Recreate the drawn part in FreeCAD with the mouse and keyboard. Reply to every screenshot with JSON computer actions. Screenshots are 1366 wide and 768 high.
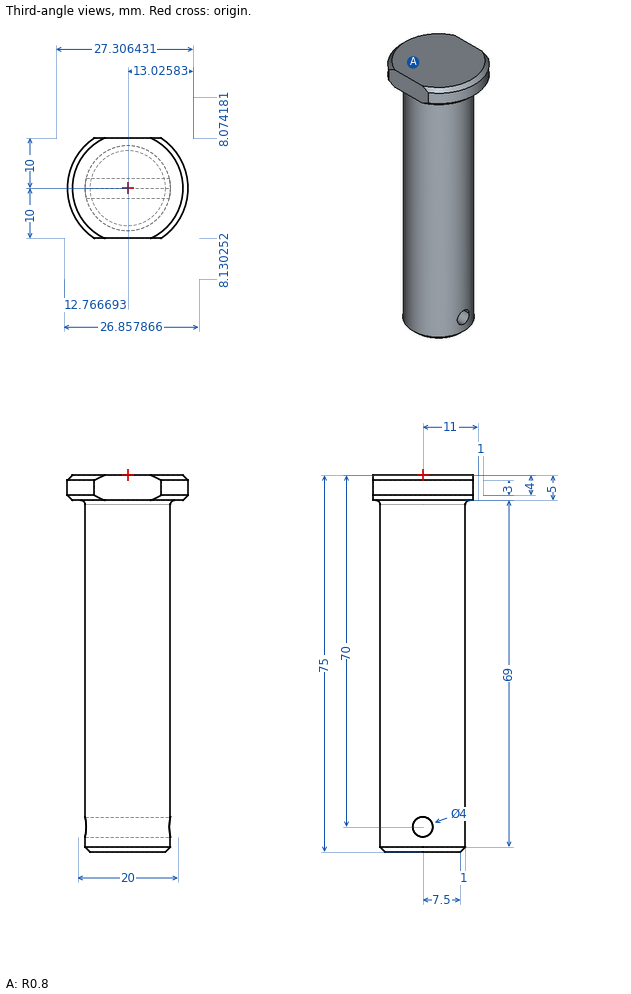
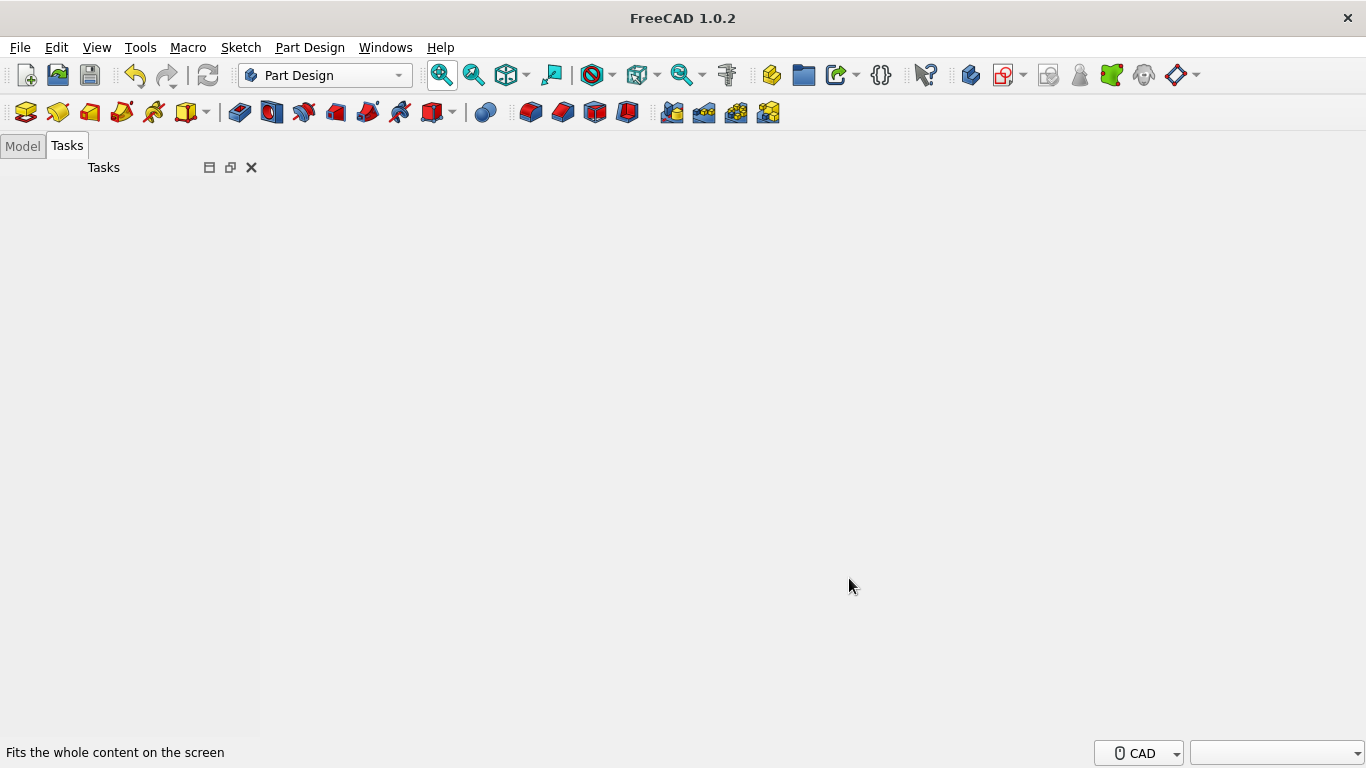
{"action": "left_click", "coordinate": [26, 76]}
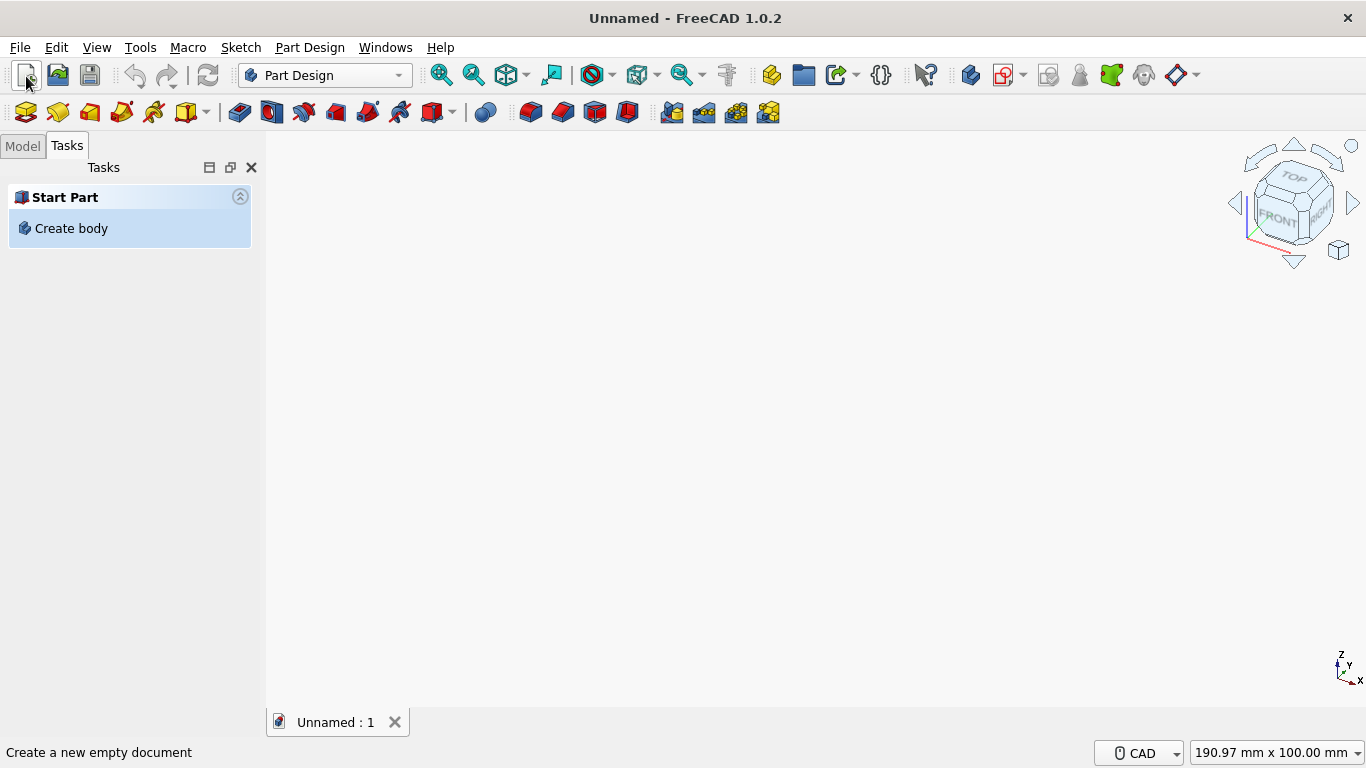
{"action": "left_click", "coordinate": [1004, 76]}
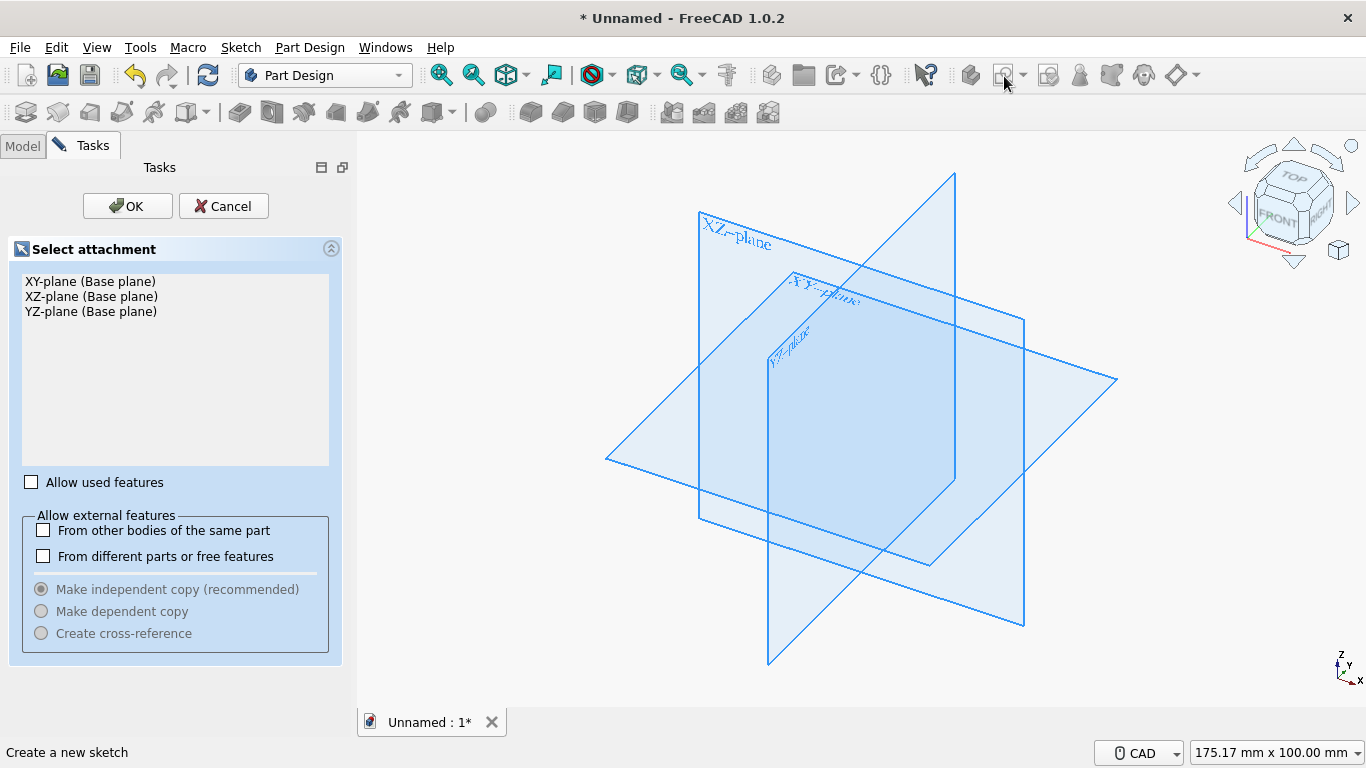
{"action": "left_click", "coordinate": [82, 312]}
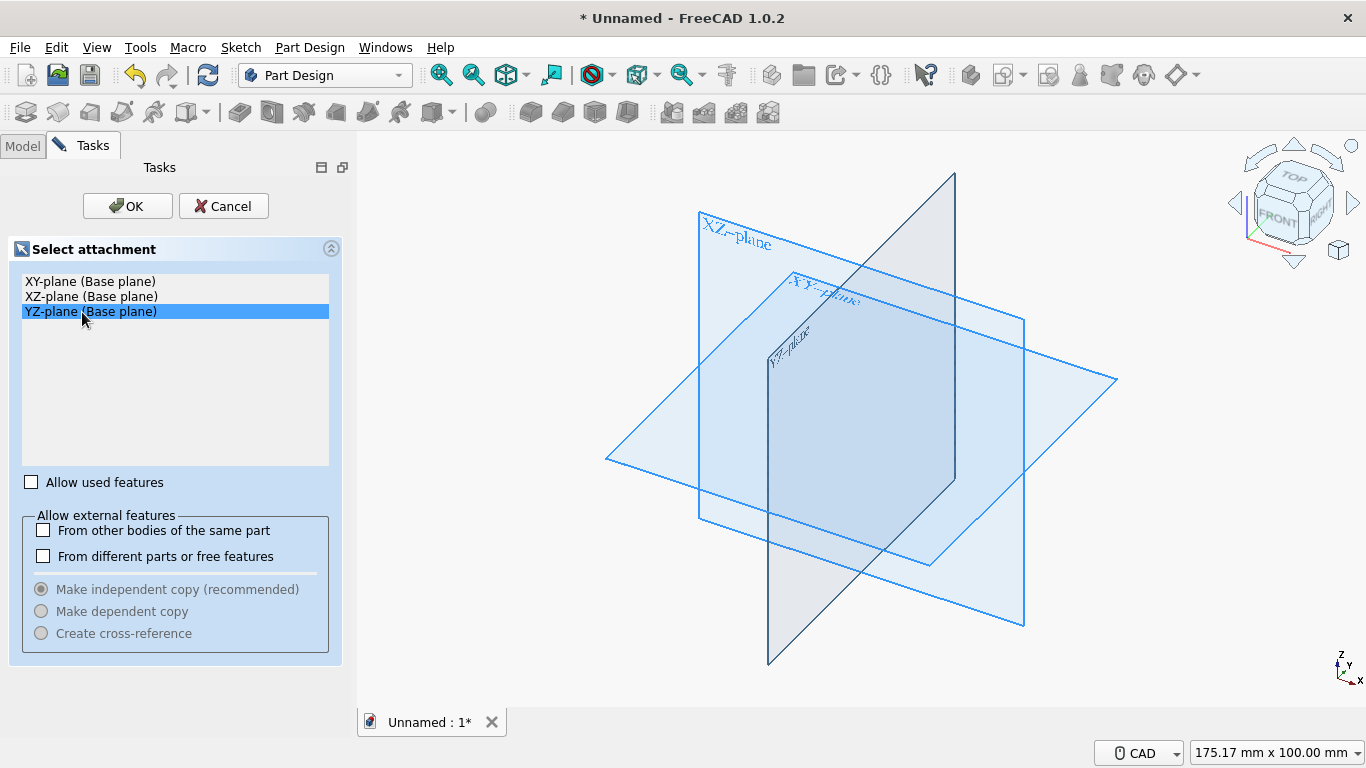
{"action": "left_click", "coordinate": [128, 206]}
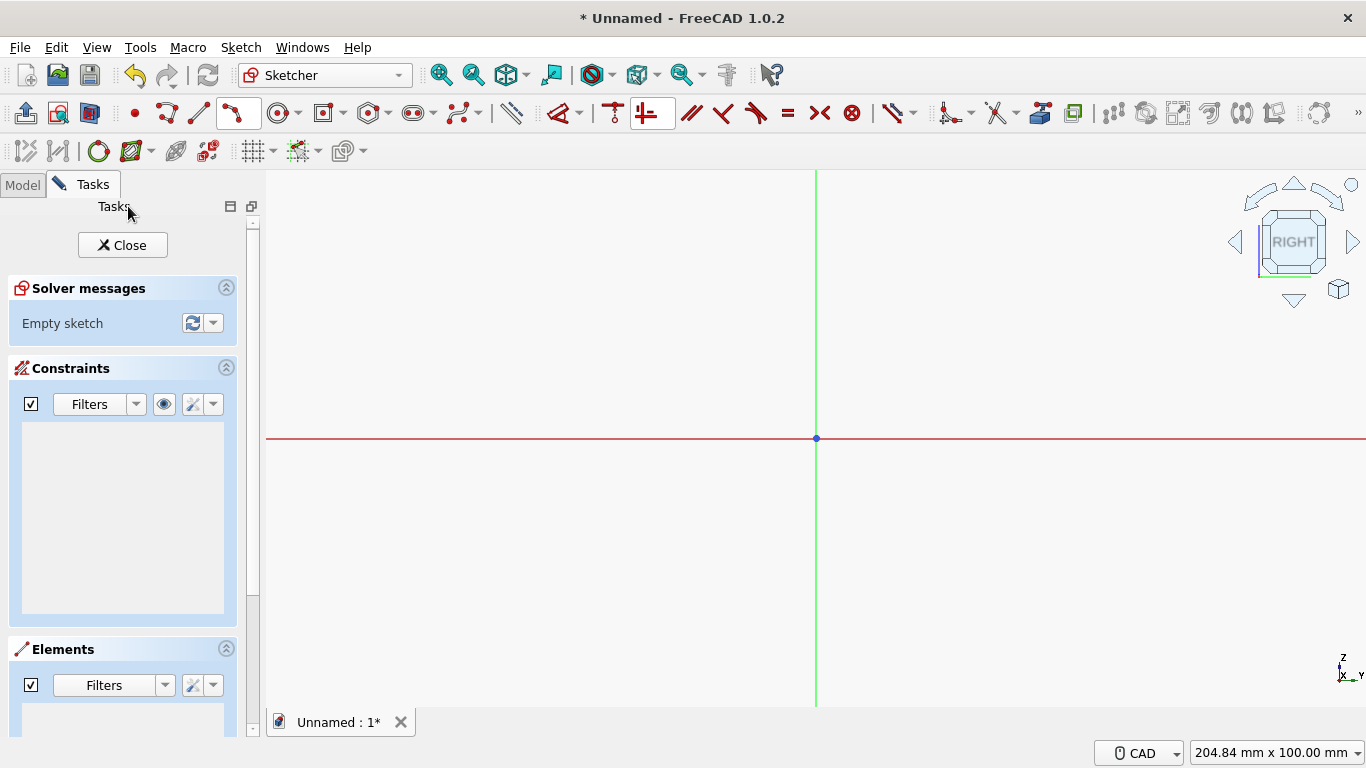
{"action": "scroll", "coordinate": [543, 198], "scroll_direction": "down", "scroll_amount": 2}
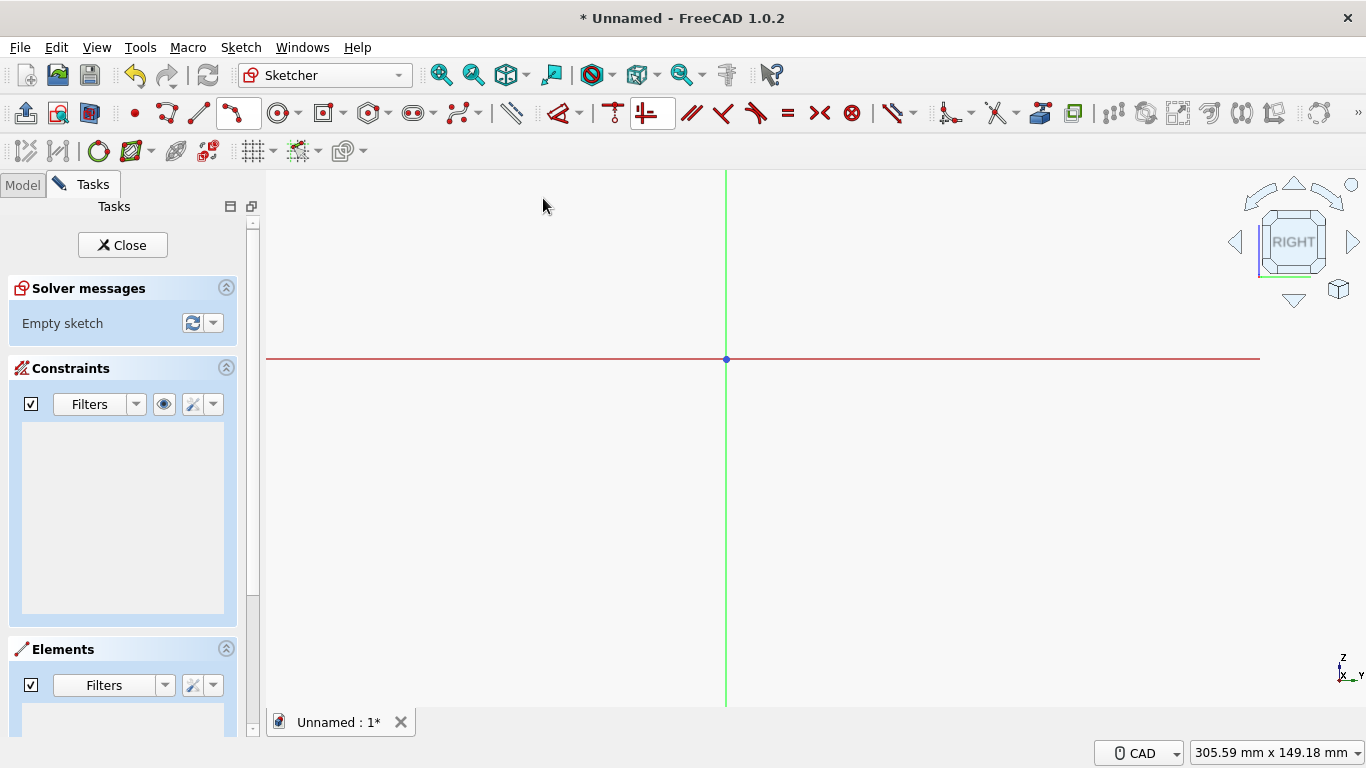
{"action": "left_click", "coordinate": [168, 114]}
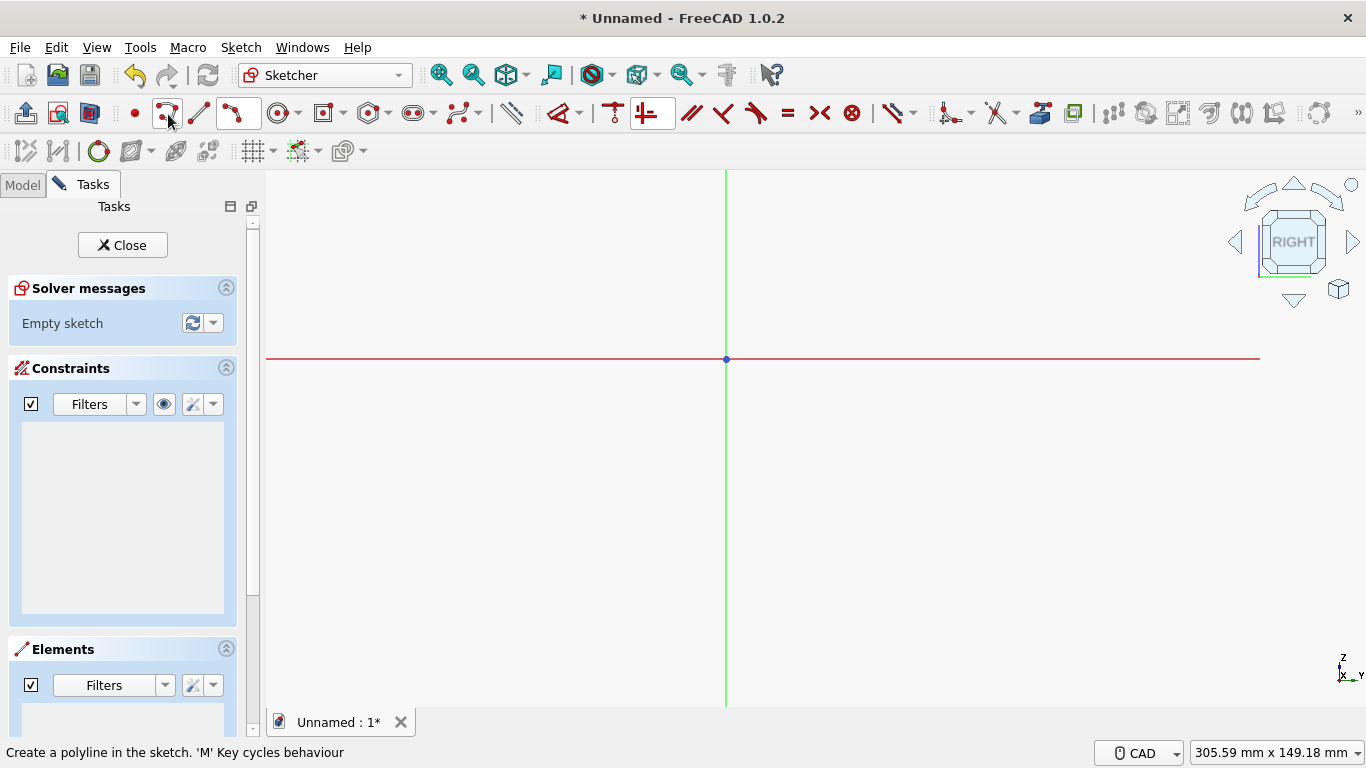
{"action": "left_click", "coordinate": [726, 359]}
{"action": "left_click", "coordinate": [735, 629]}
{"action": "left_click", "coordinate": [753, 629]}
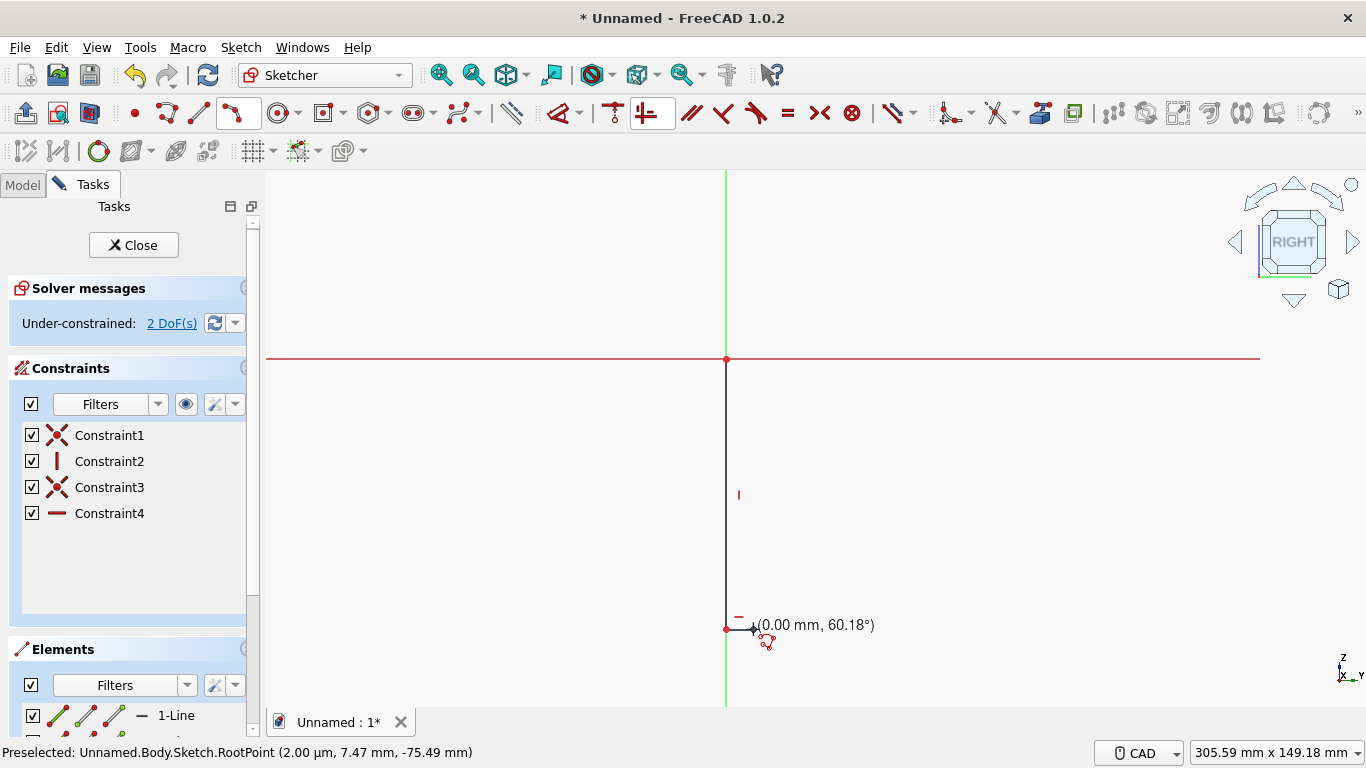
{"action": "scroll", "coordinate": [757, 626], "scroll_direction": "up", "scroll_amount": 6}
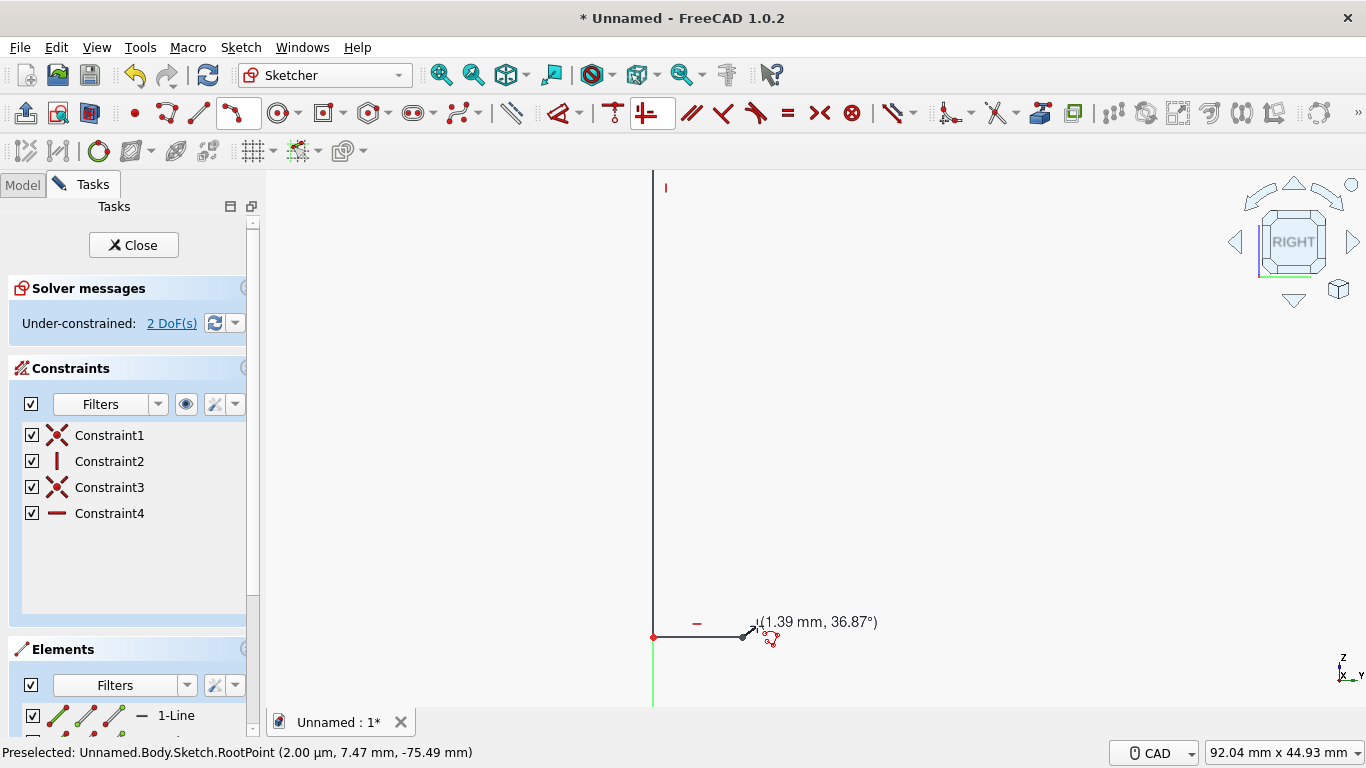
{"action": "left_click", "coordinate": [755, 623]}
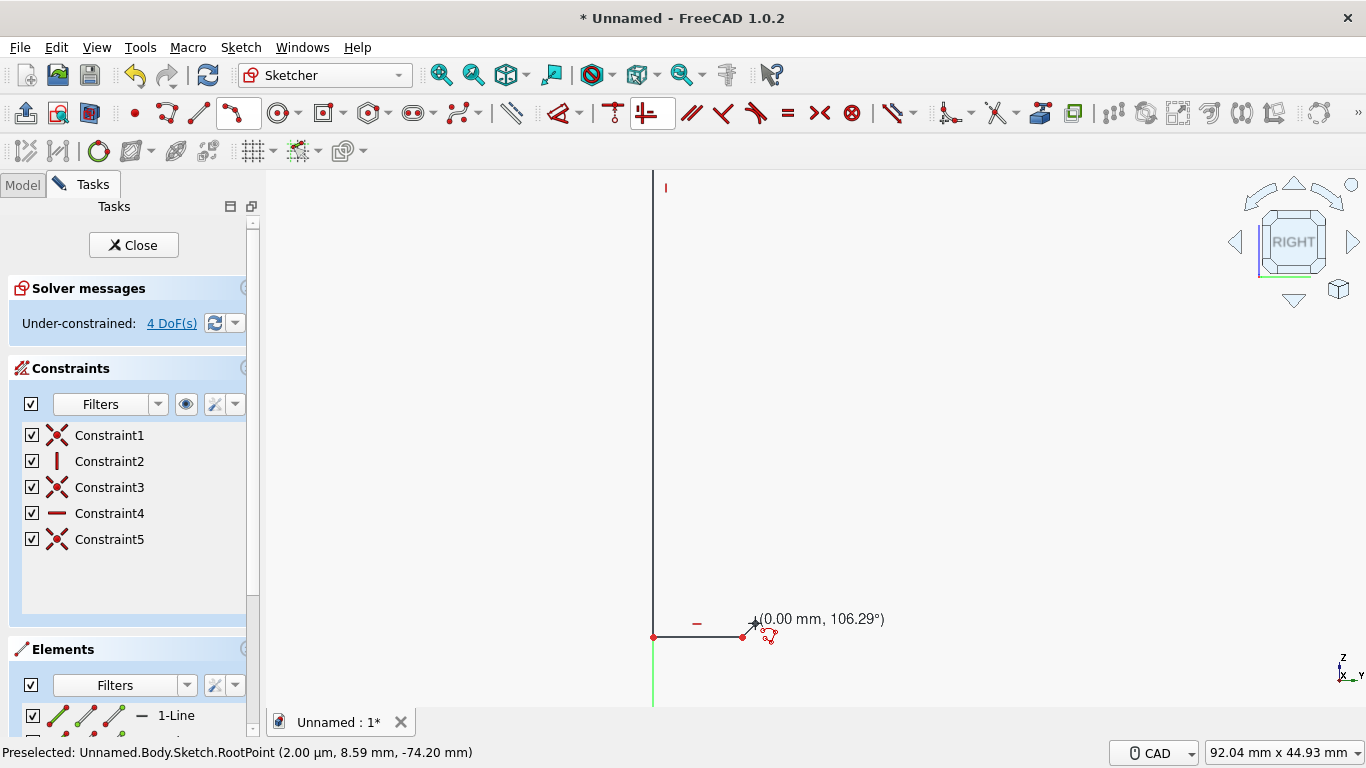
{"action": "scroll", "coordinate": [761, 585], "scroll_direction": "down", "scroll_amount": 5}